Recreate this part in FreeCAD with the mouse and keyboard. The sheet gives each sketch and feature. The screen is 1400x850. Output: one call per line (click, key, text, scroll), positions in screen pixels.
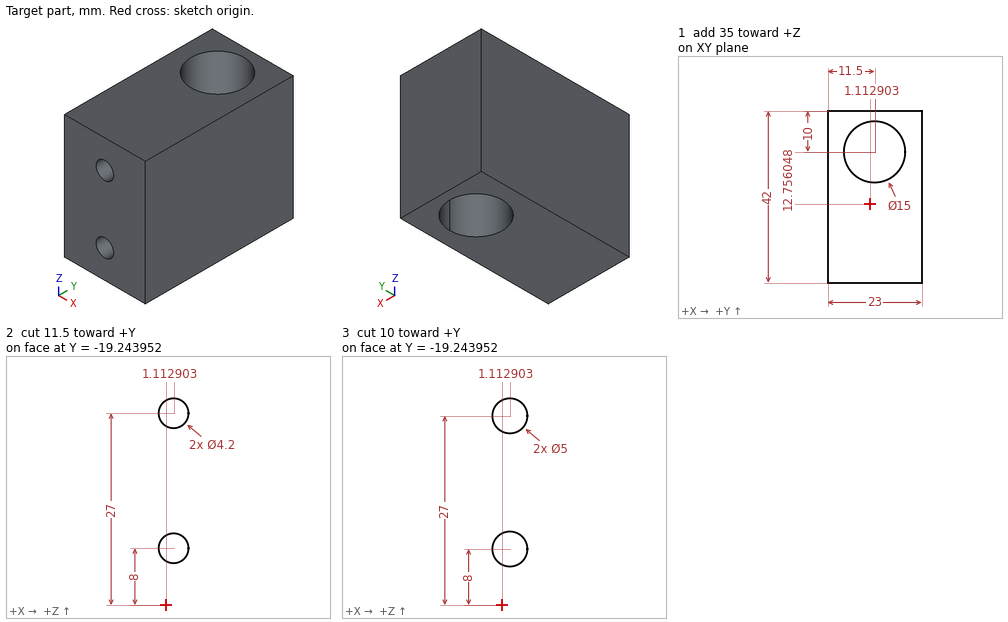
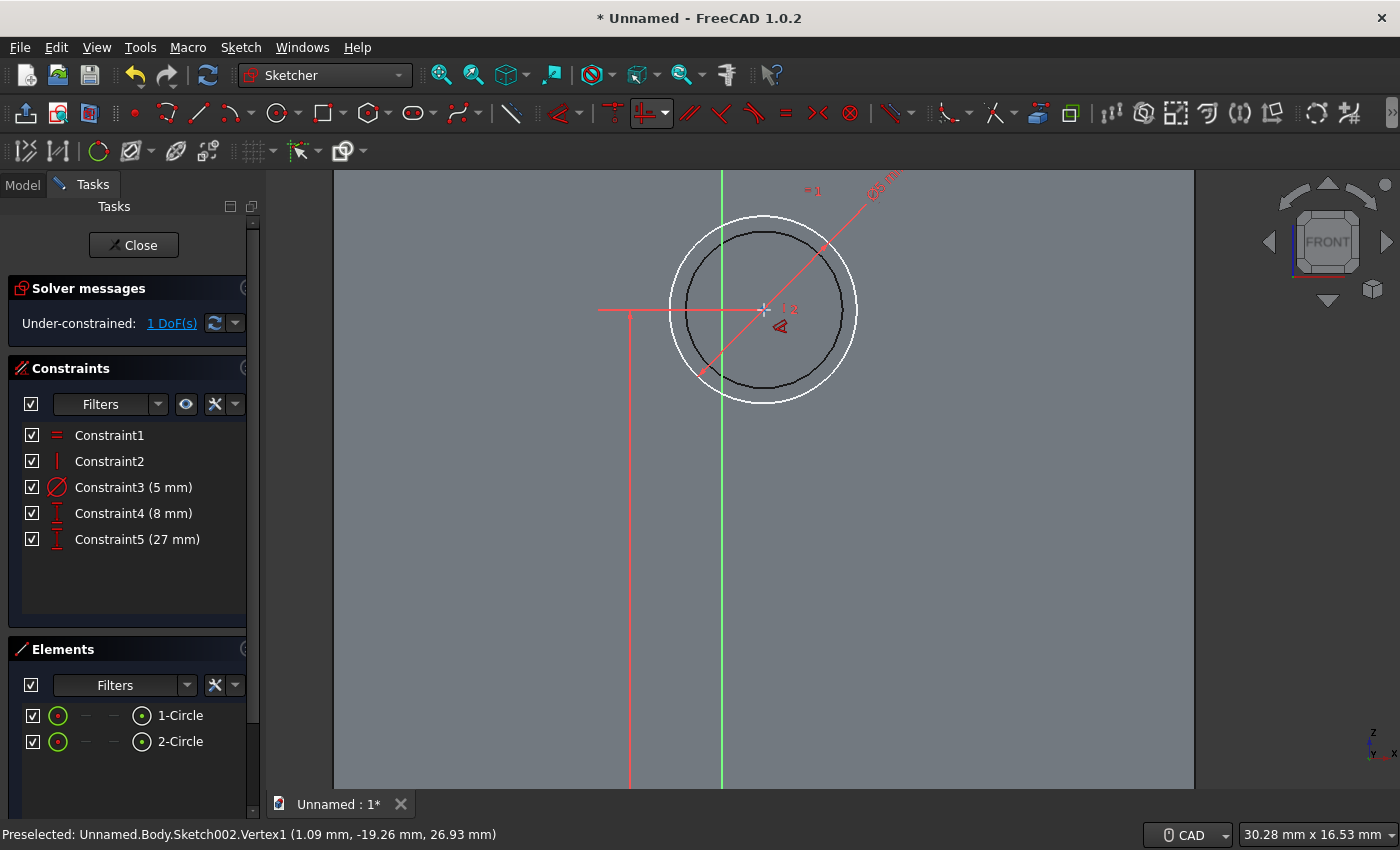
click(763, 310)
click(743, 276)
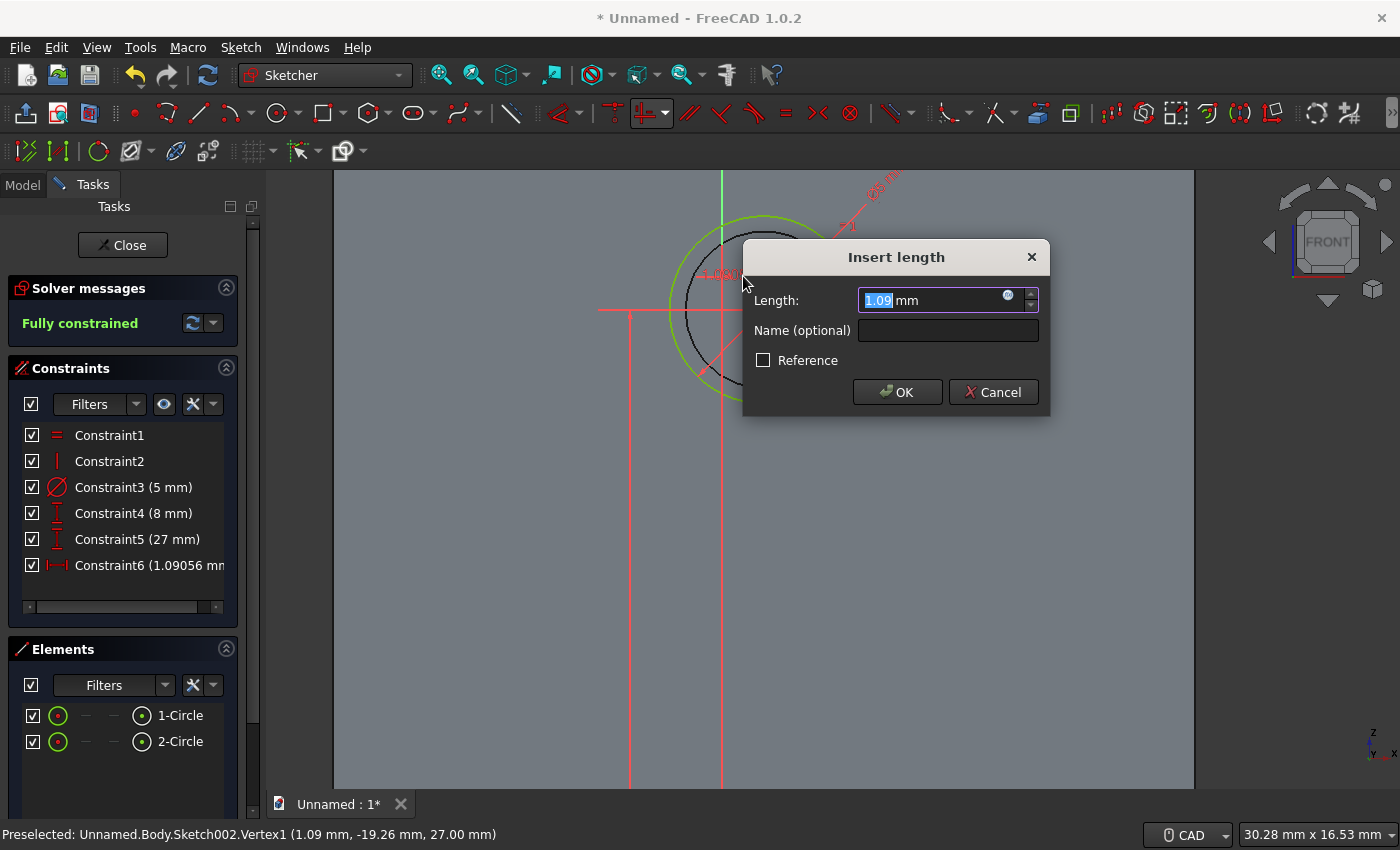
text(1.112903)
key(Return)
key(Escape)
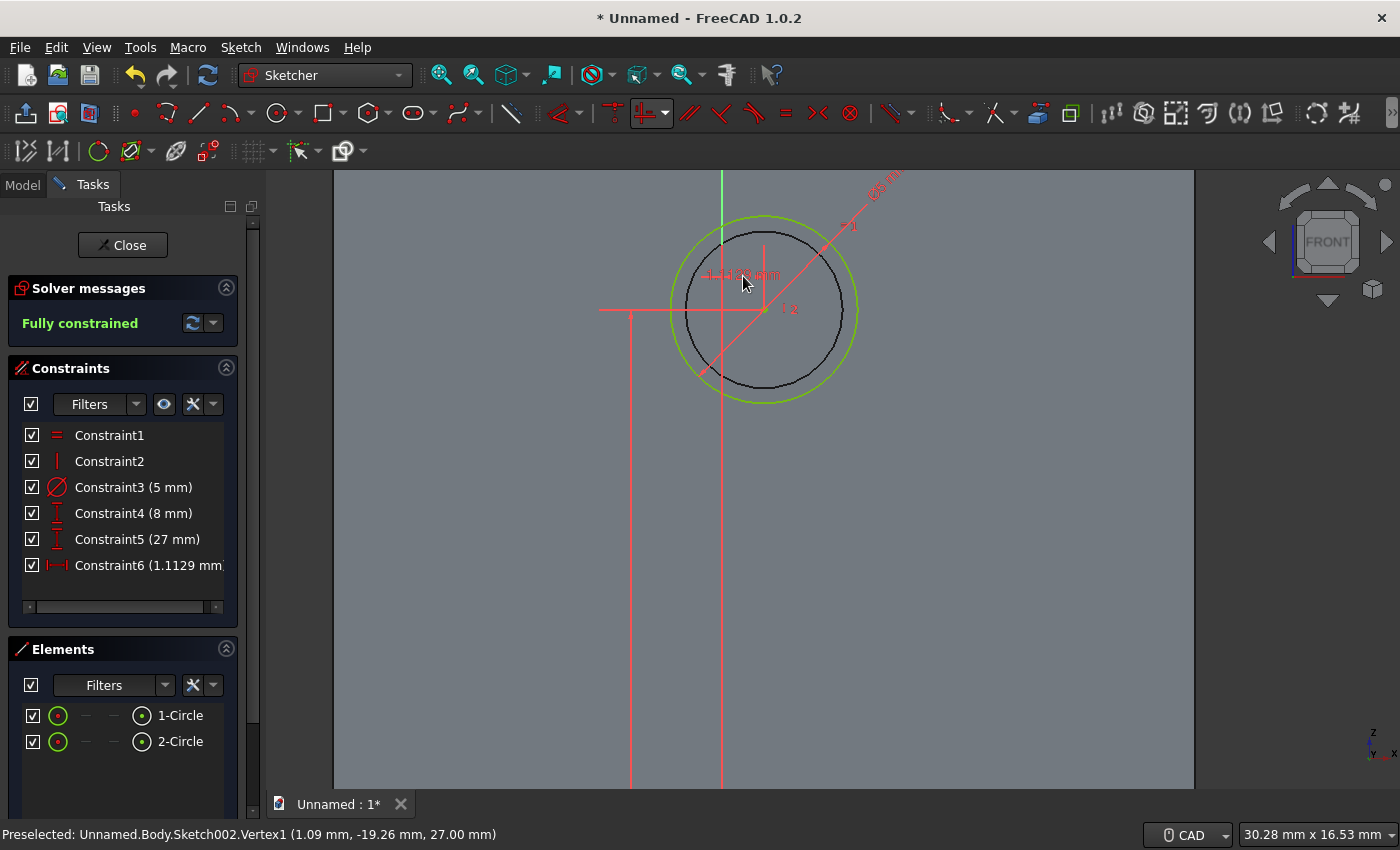
click(123, 245)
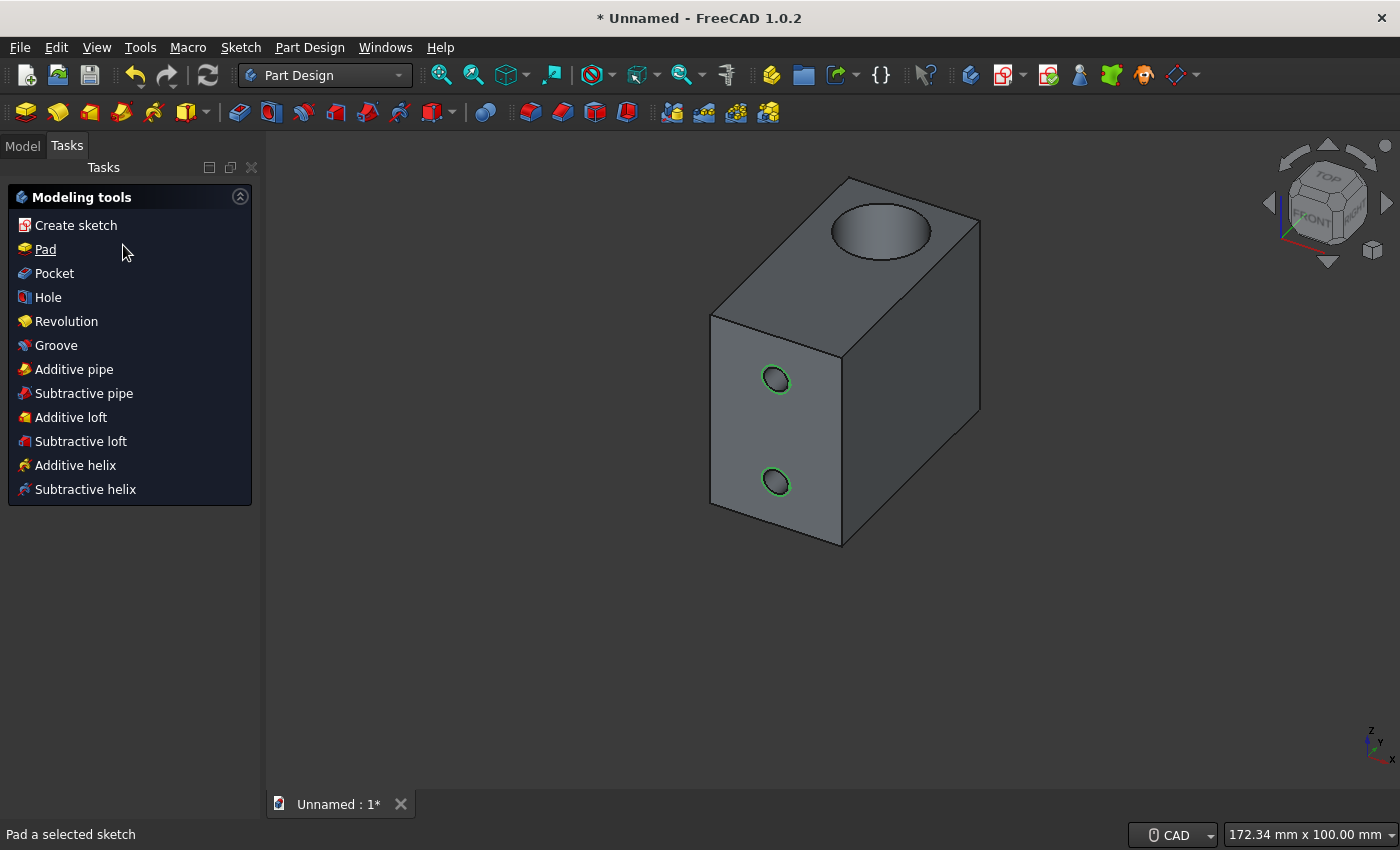
click(240, 112)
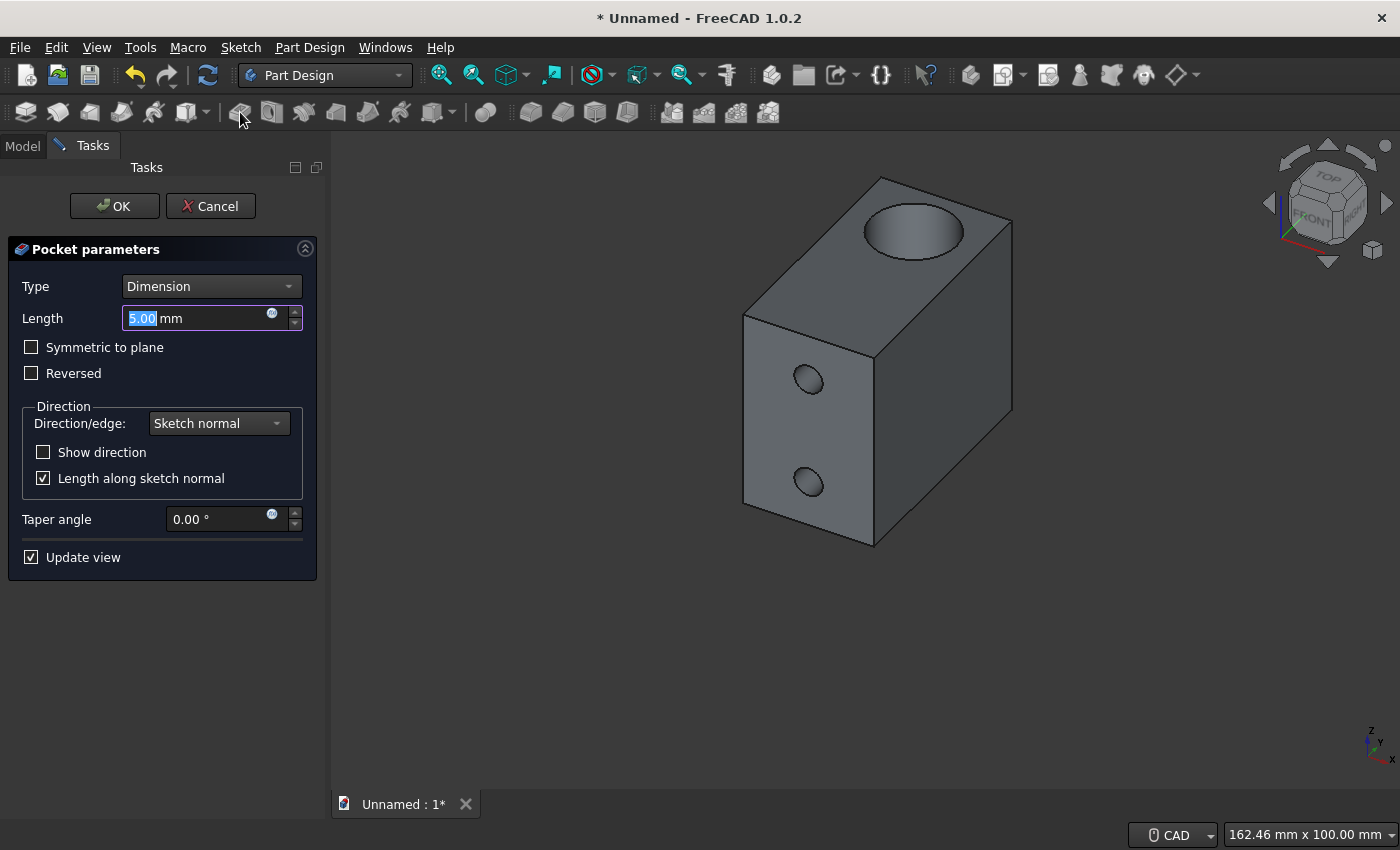
text(10)
key(Tab)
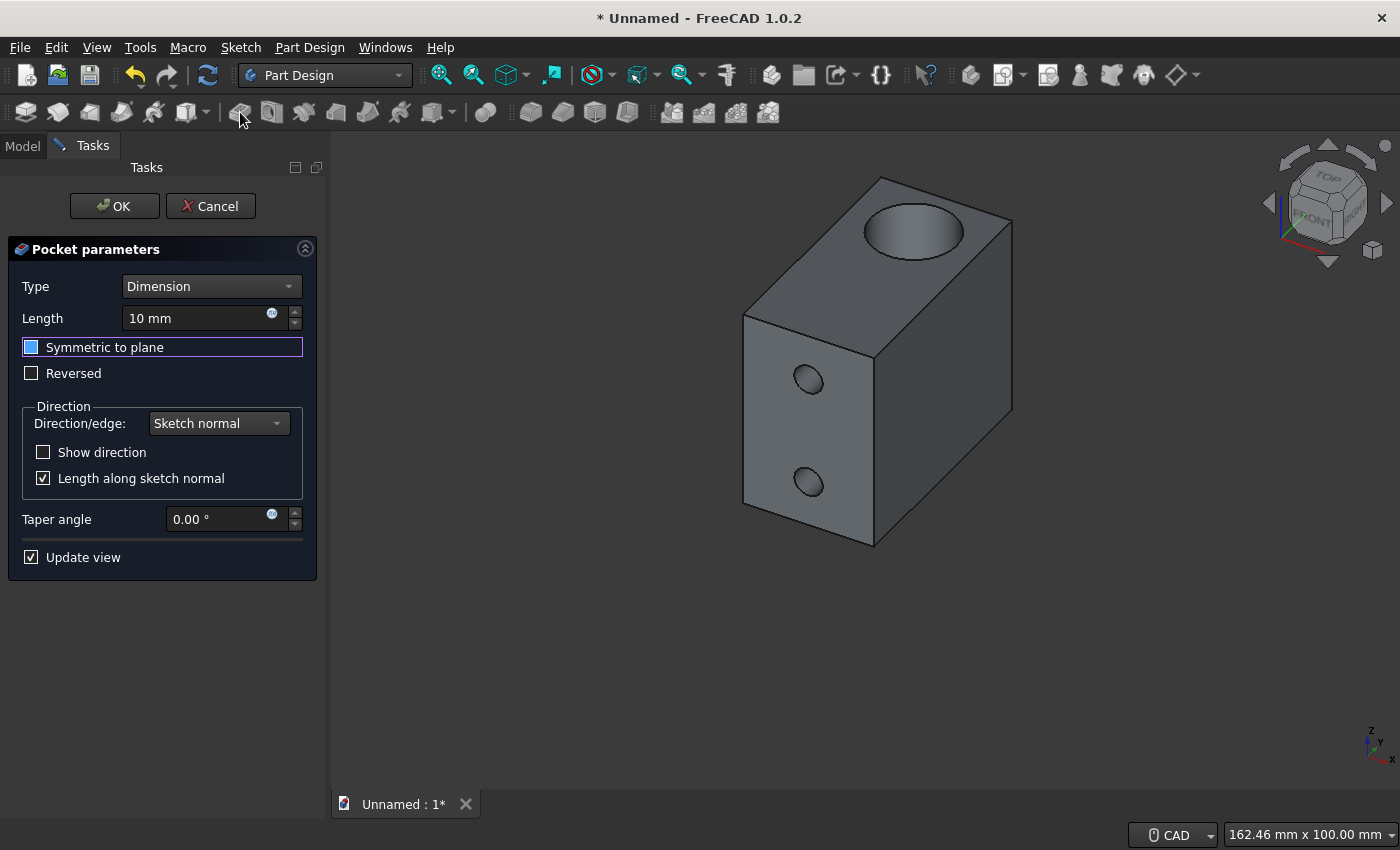
click(115, 206)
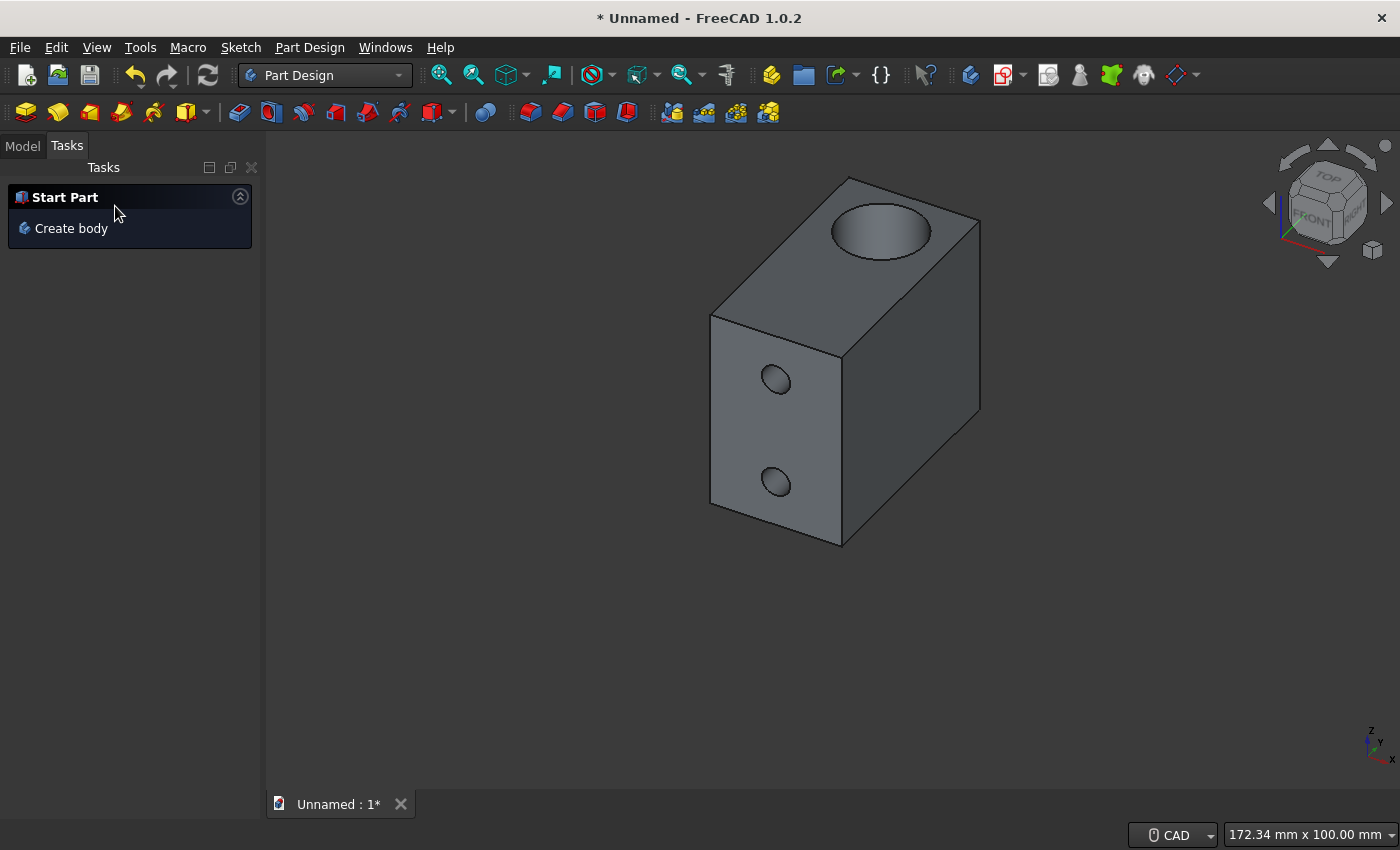
key(0)